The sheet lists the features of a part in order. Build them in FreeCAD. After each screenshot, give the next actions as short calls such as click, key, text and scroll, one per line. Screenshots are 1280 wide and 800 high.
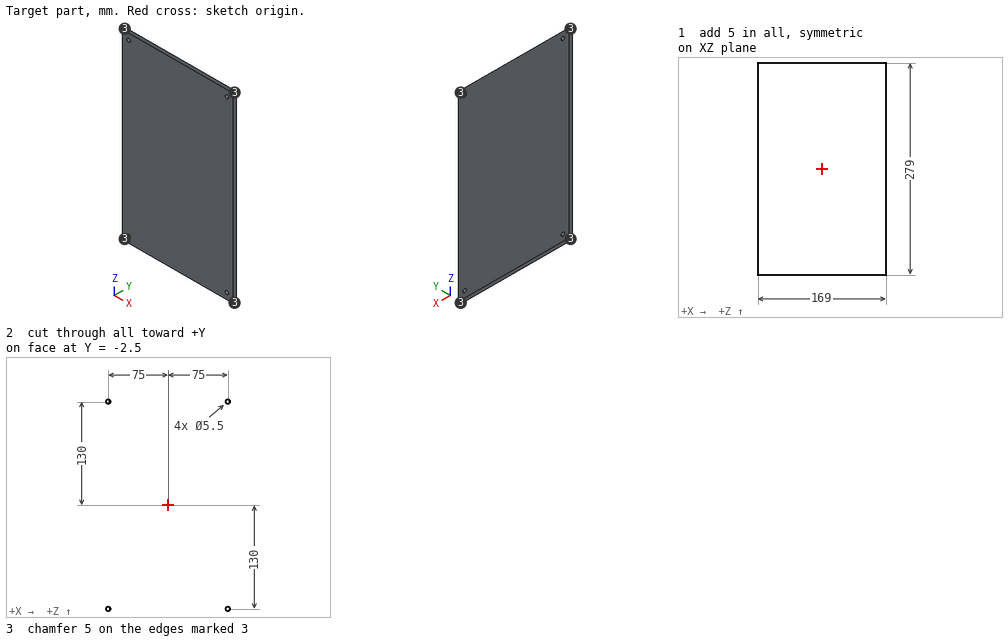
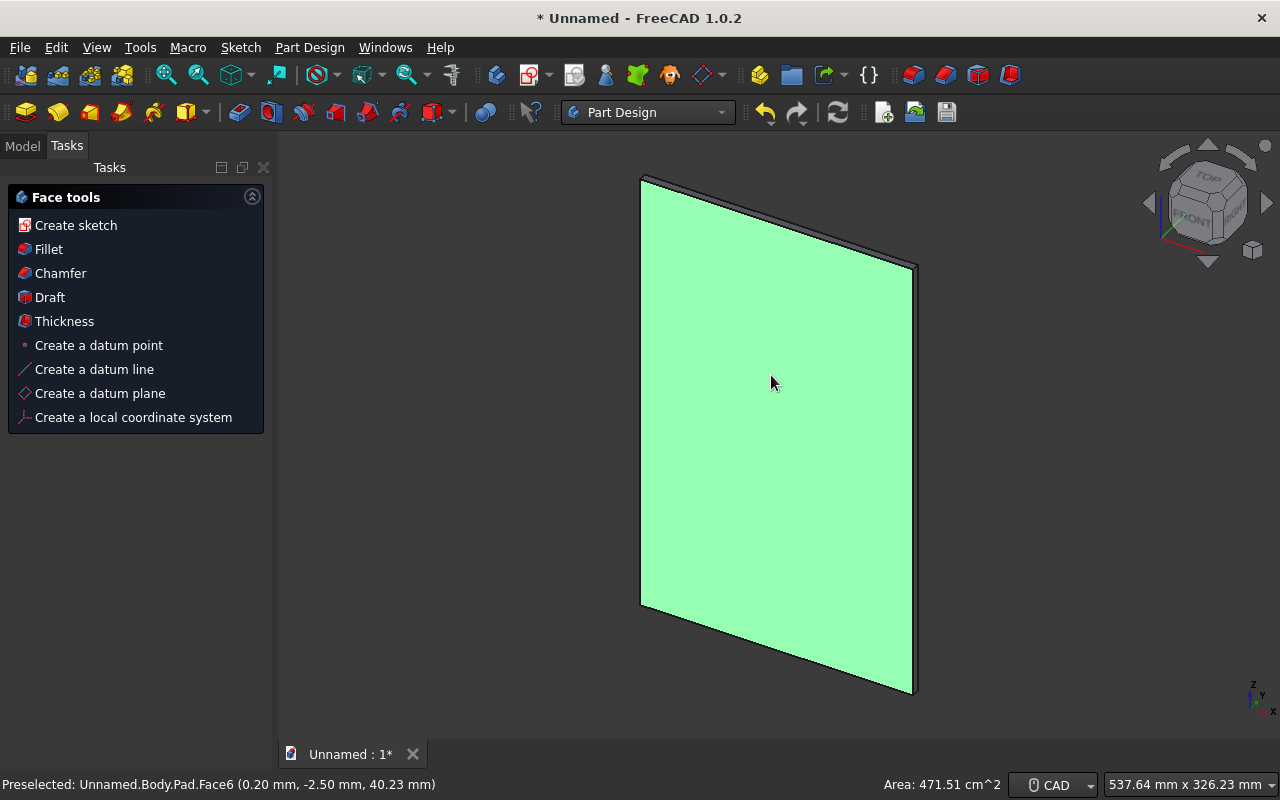
click(530, 76)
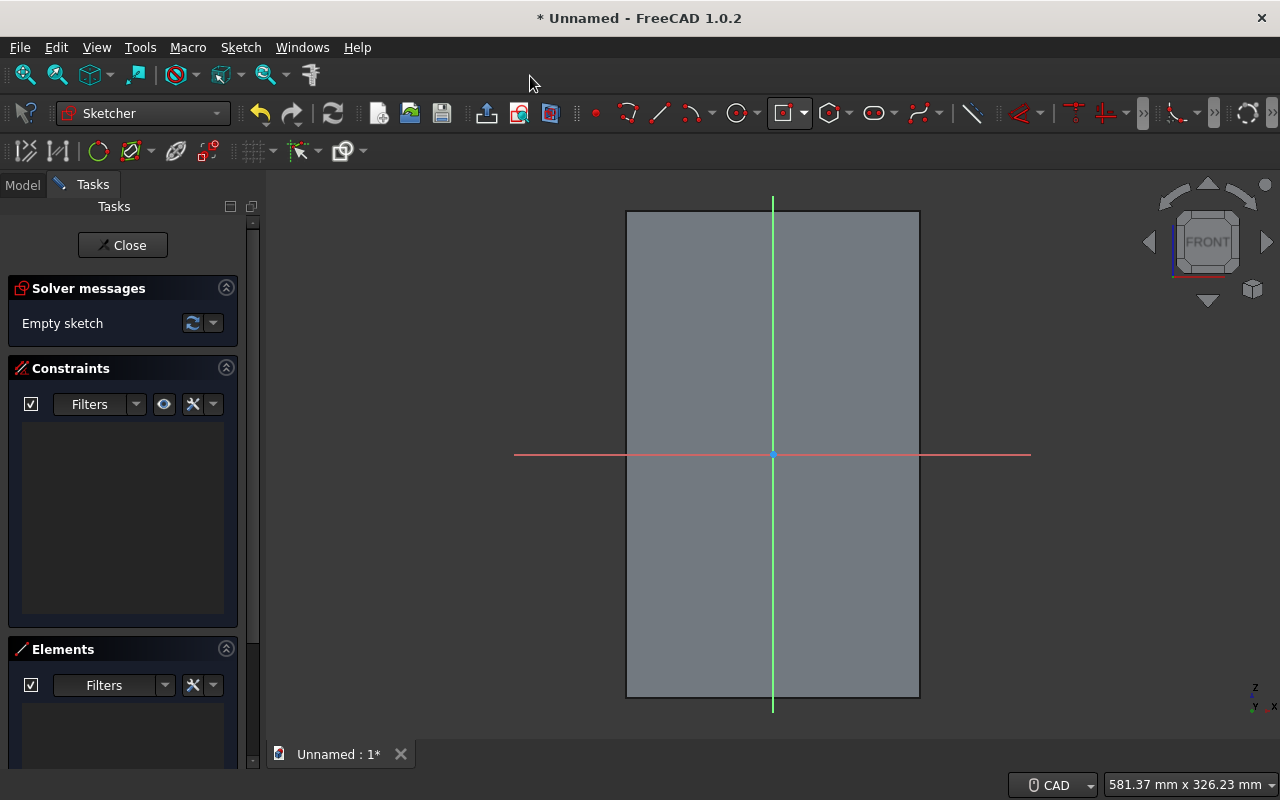
scroll(395, 455, down, 1)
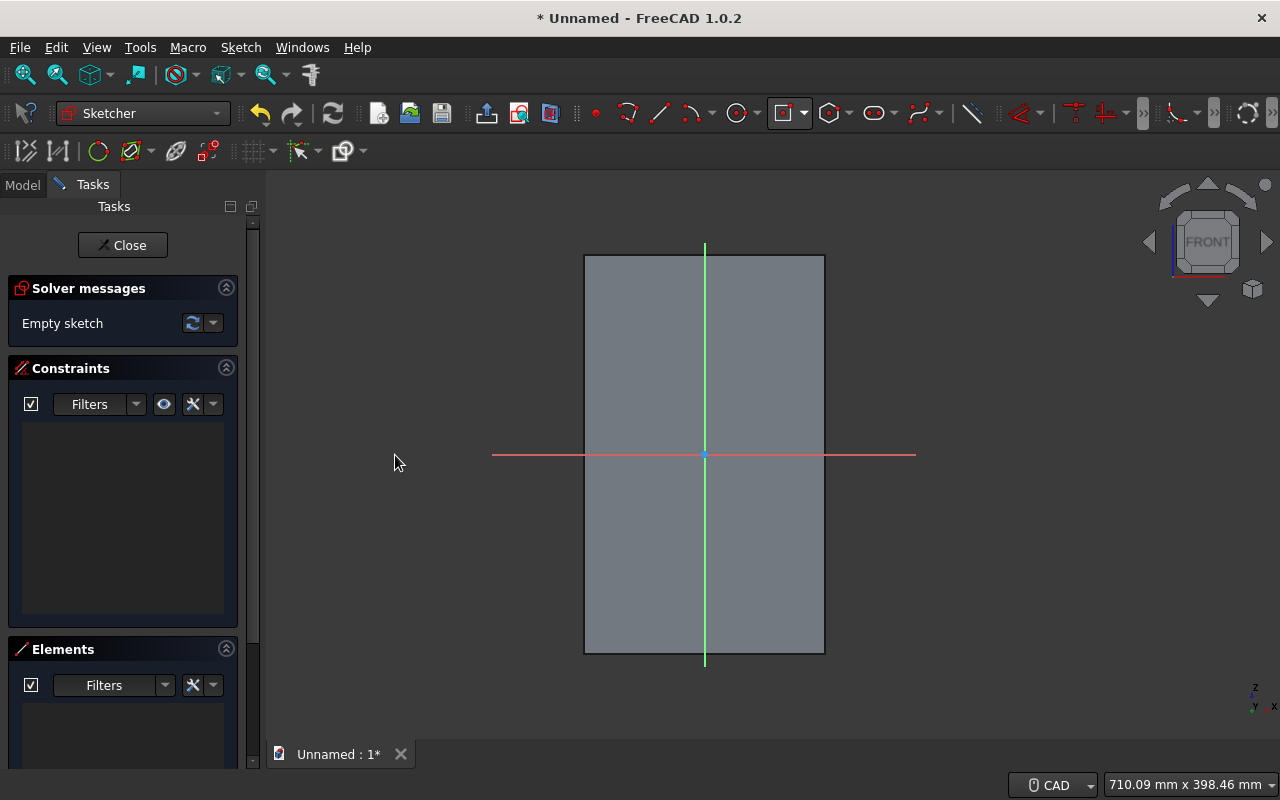
click(738, 114)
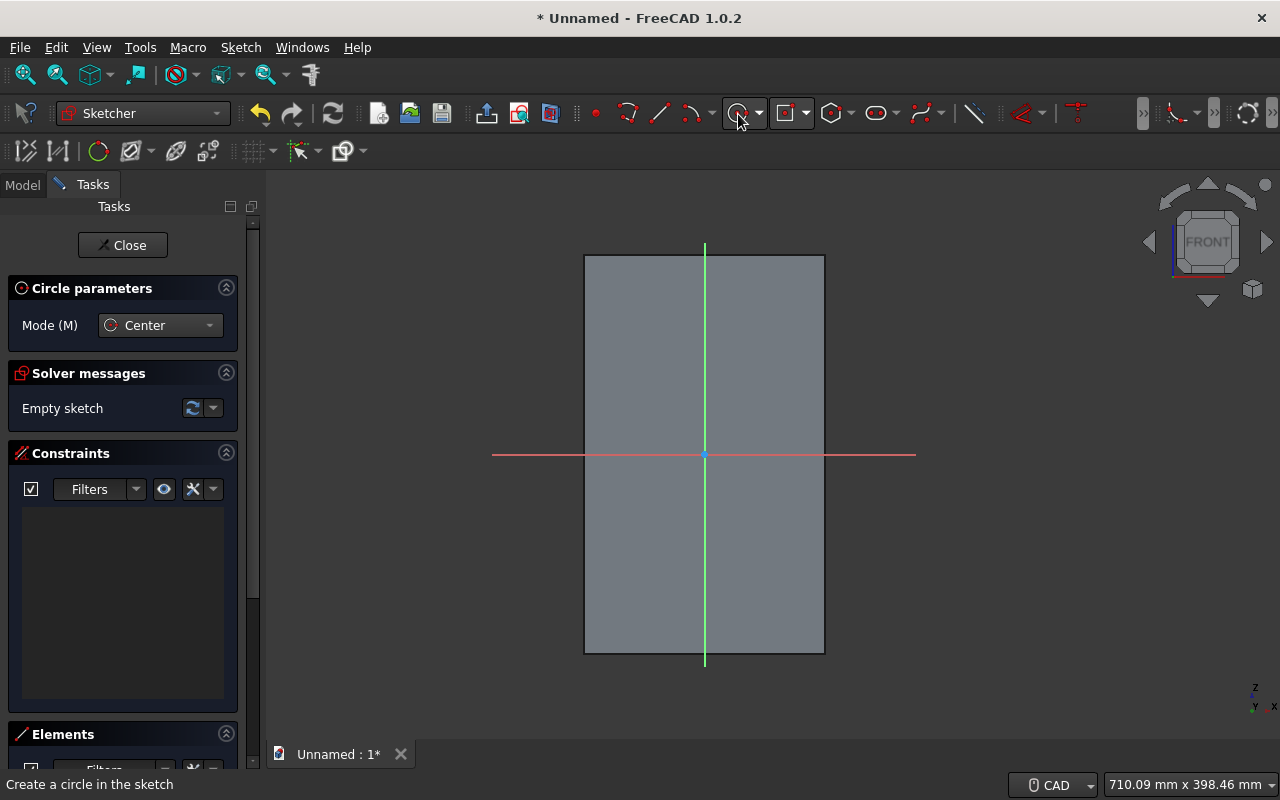
scroll(597, 269, up, 9)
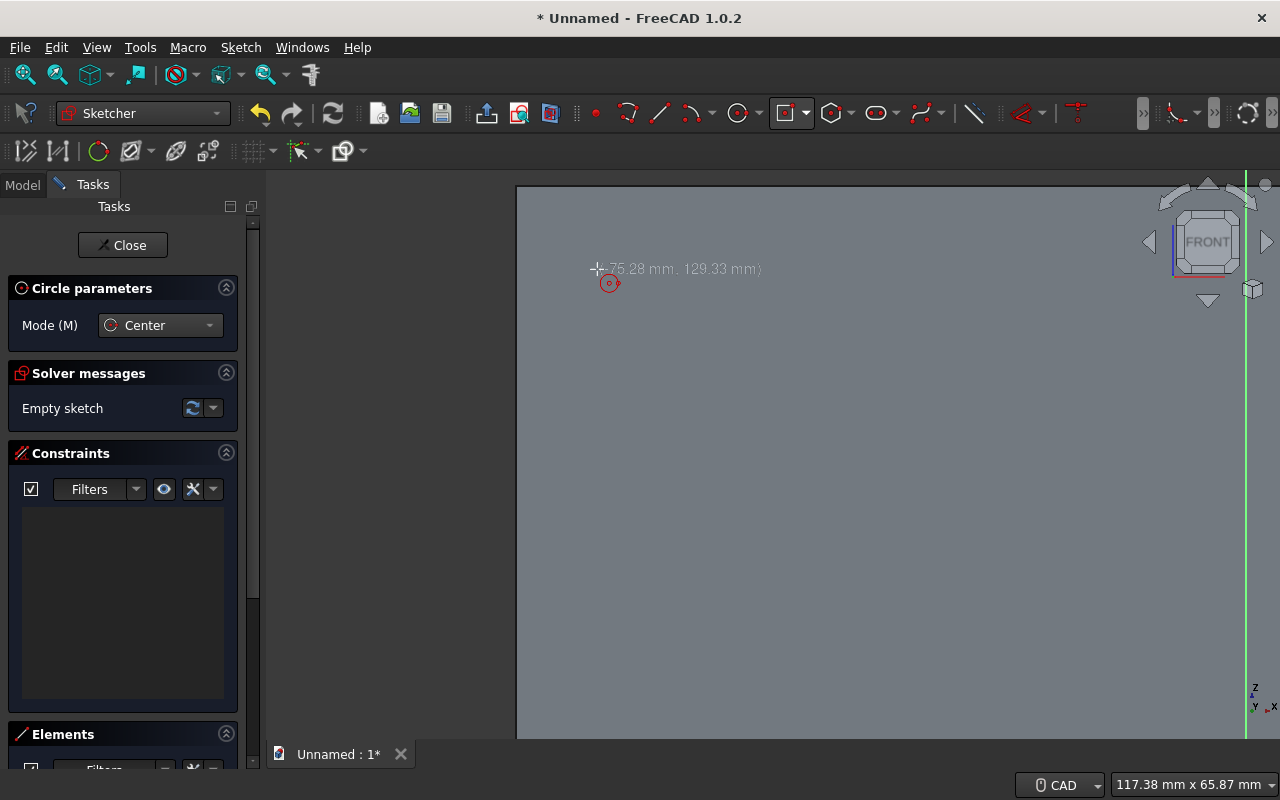
scroll(597, 269, down, 9)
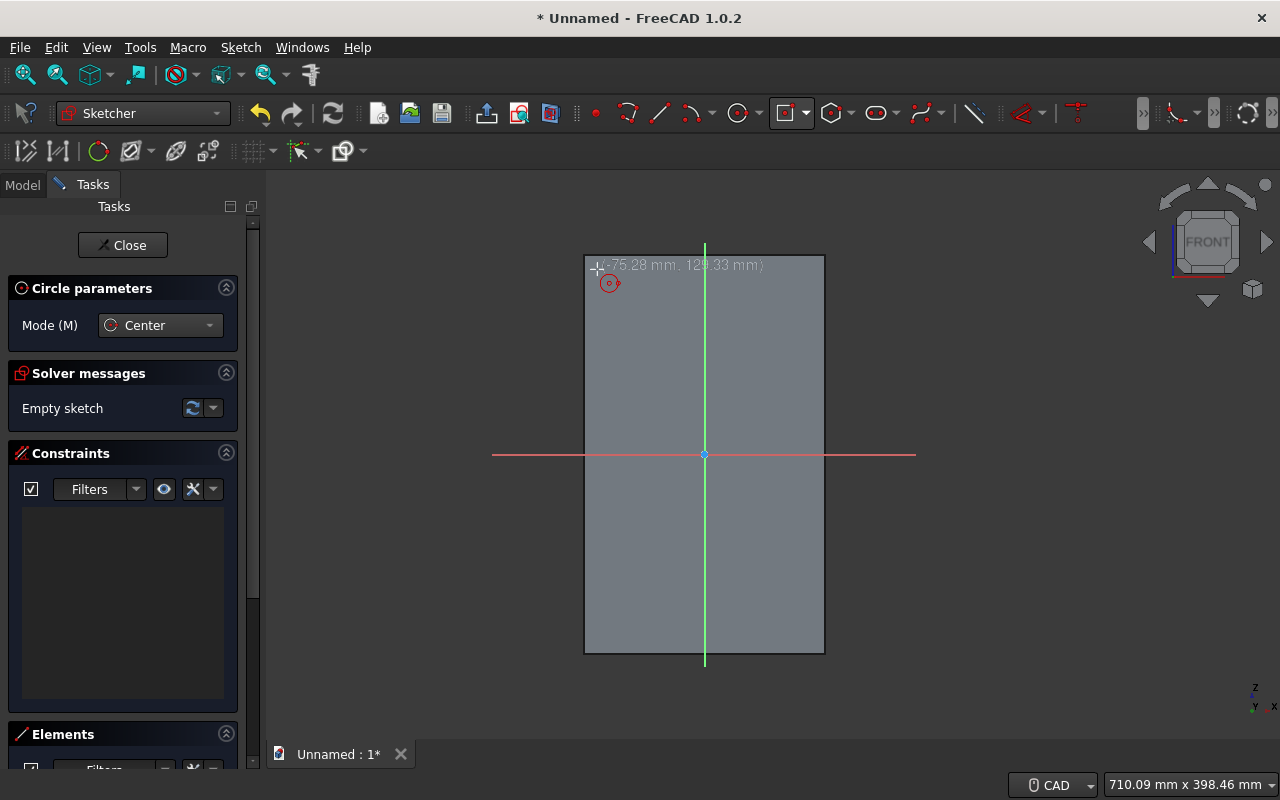
click(597, 269)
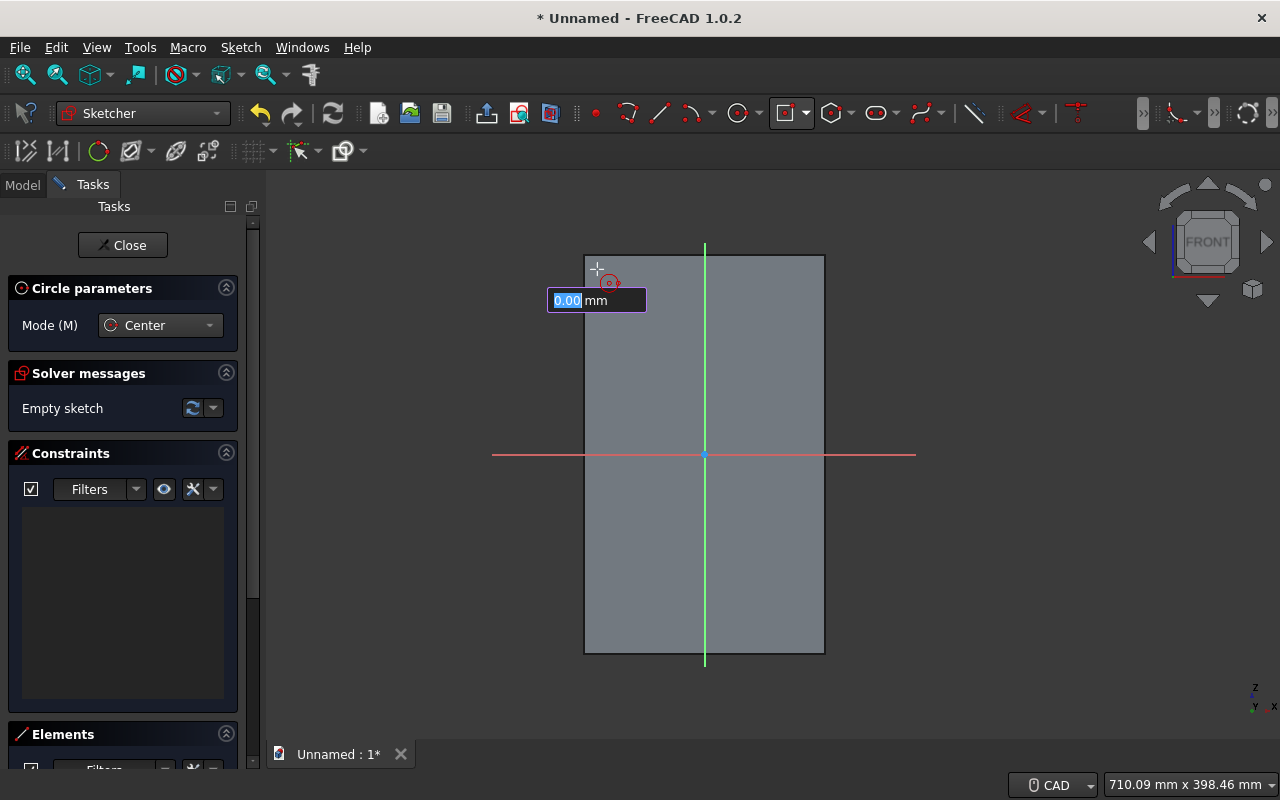
scroll(600, 266, up, 7)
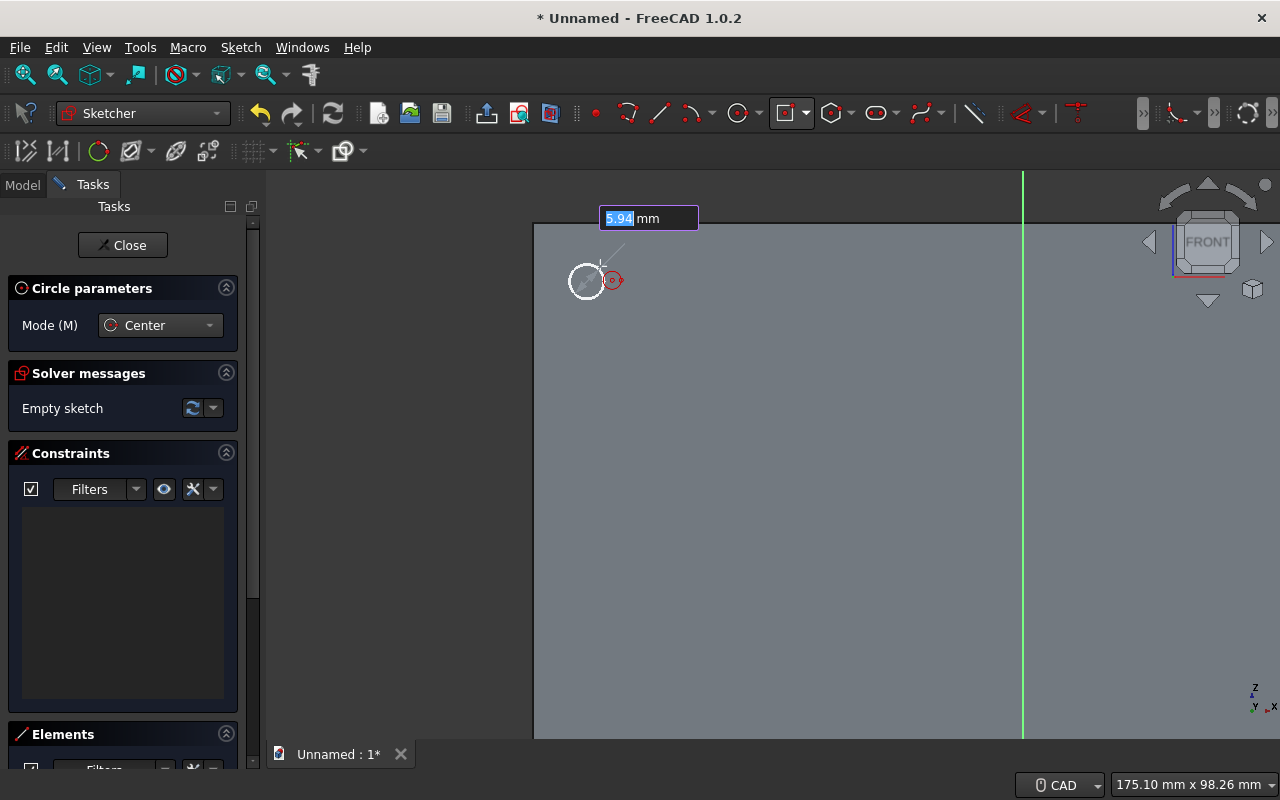
click(600, 267)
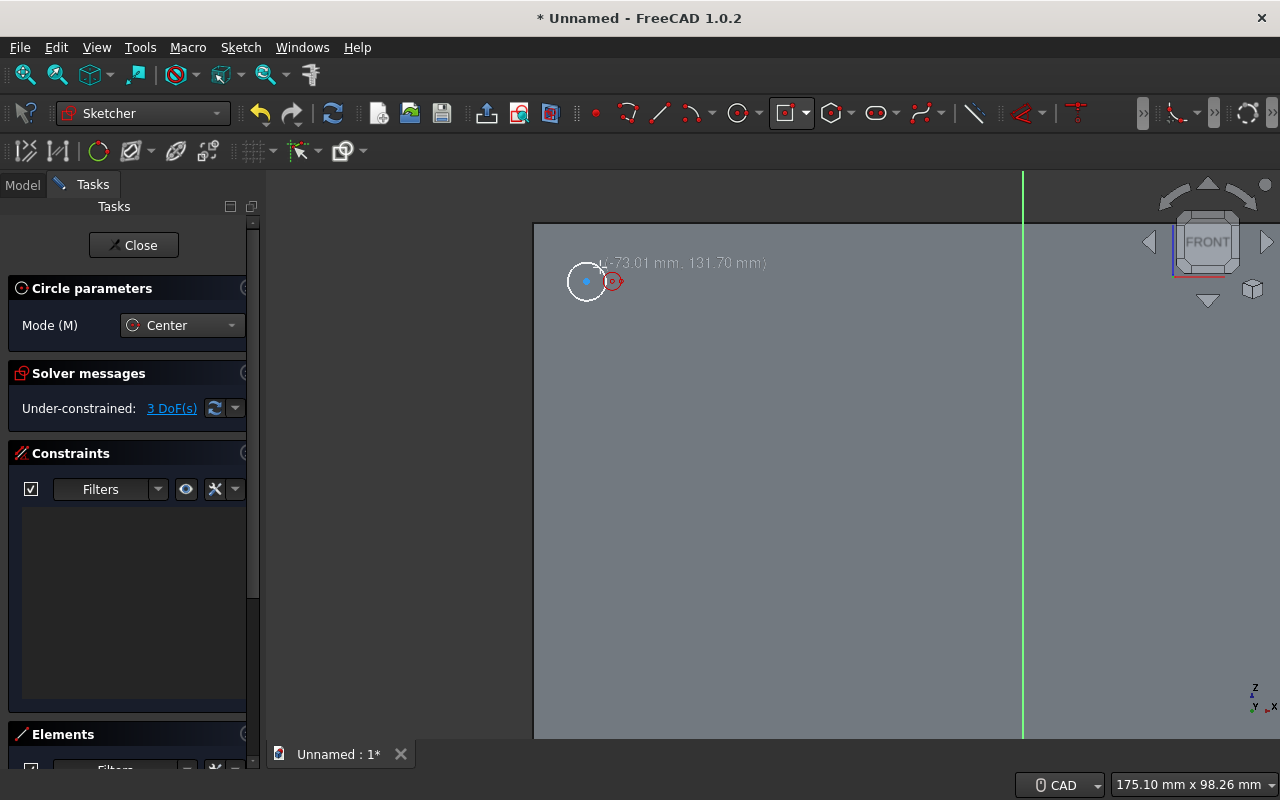
scroll(600, 266, down, 7)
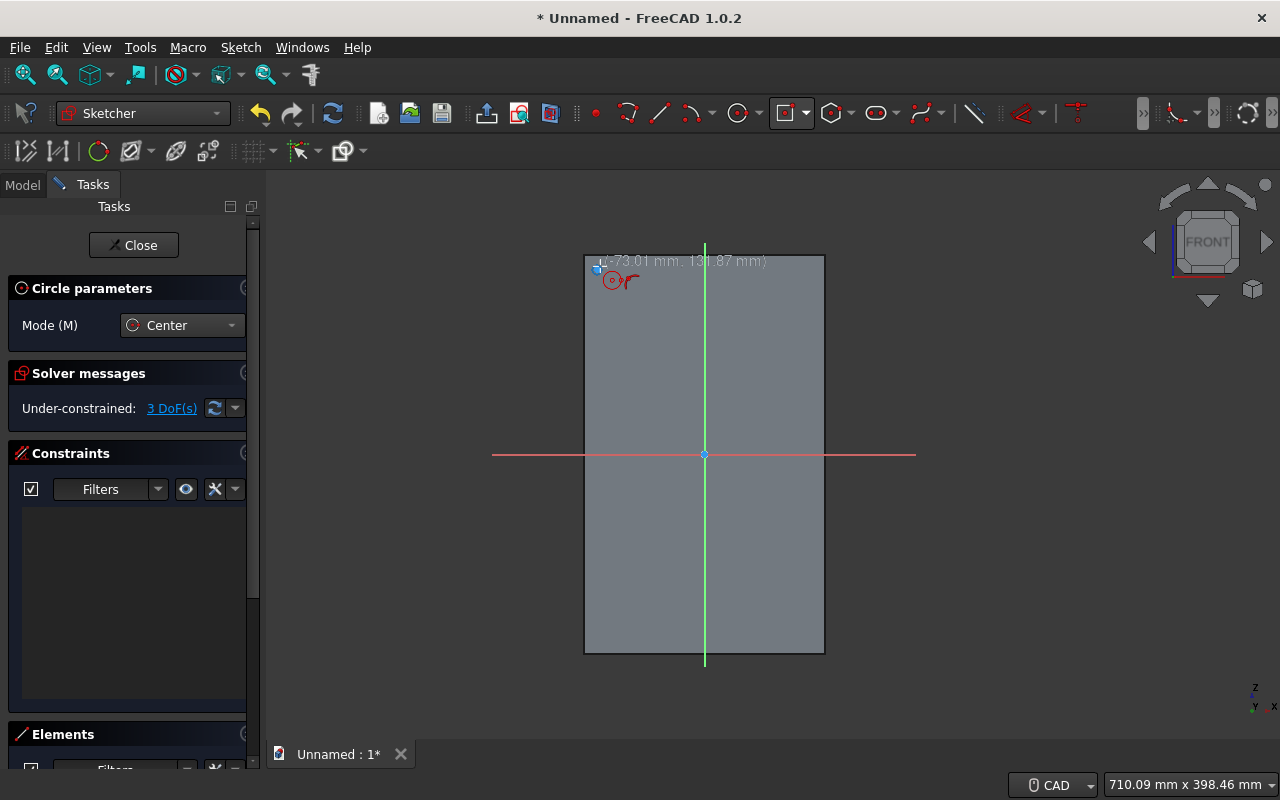
scroll(812, 269, up, 9)